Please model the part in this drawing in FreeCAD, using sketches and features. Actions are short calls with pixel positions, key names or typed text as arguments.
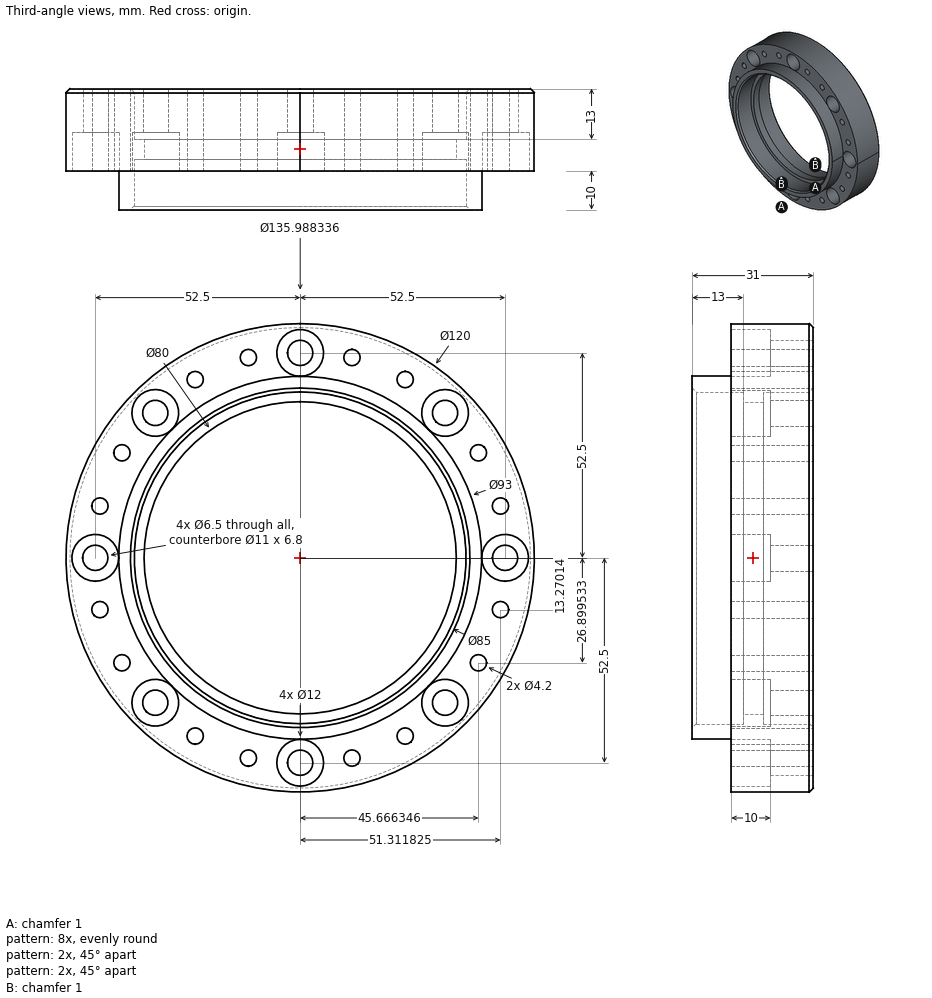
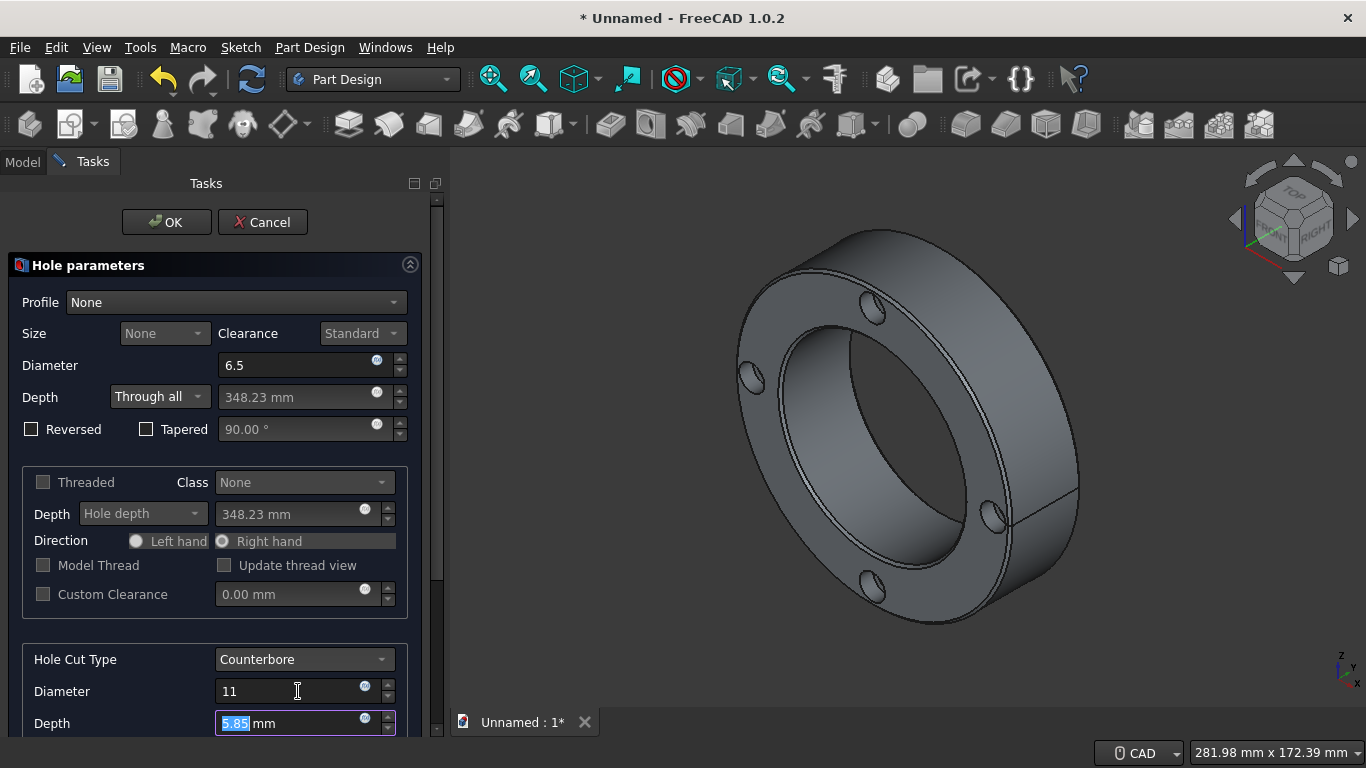
text(6.8)
key(Tab)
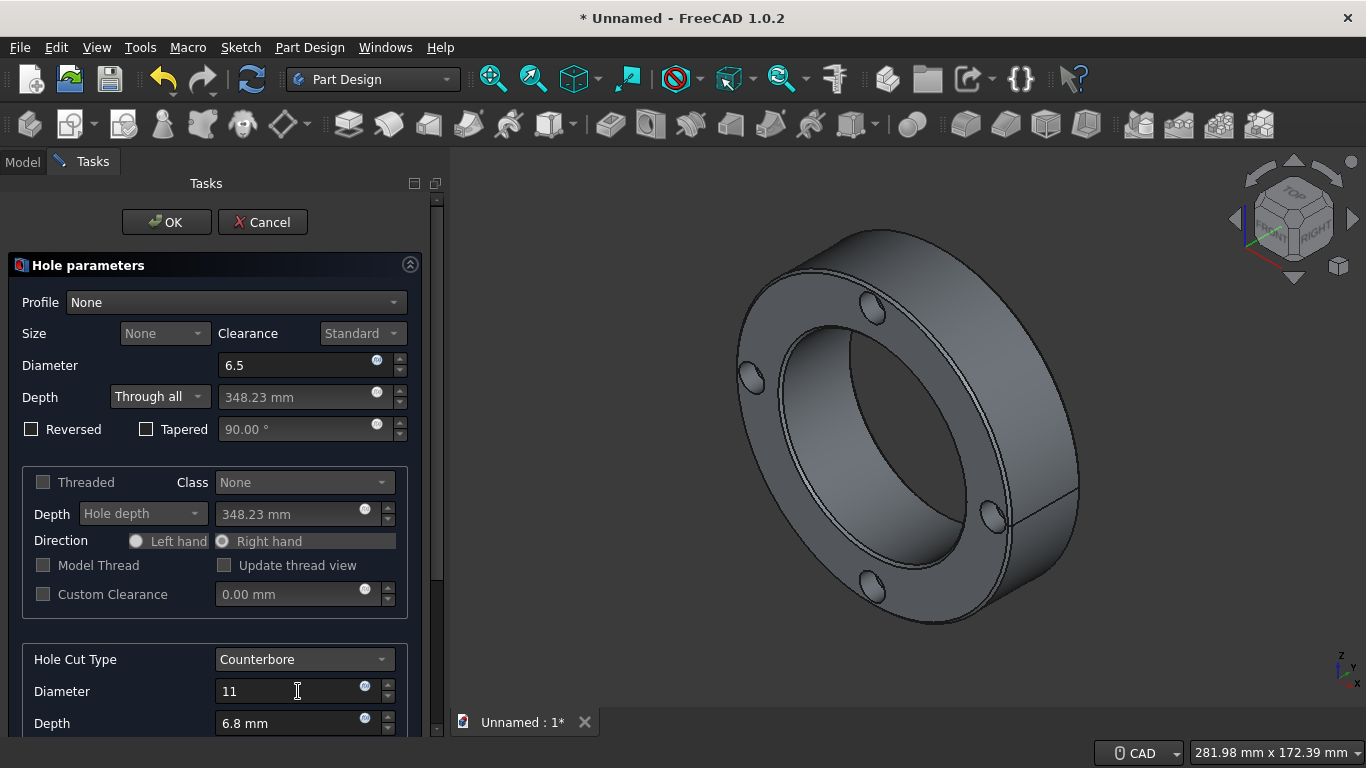
click(167, 222)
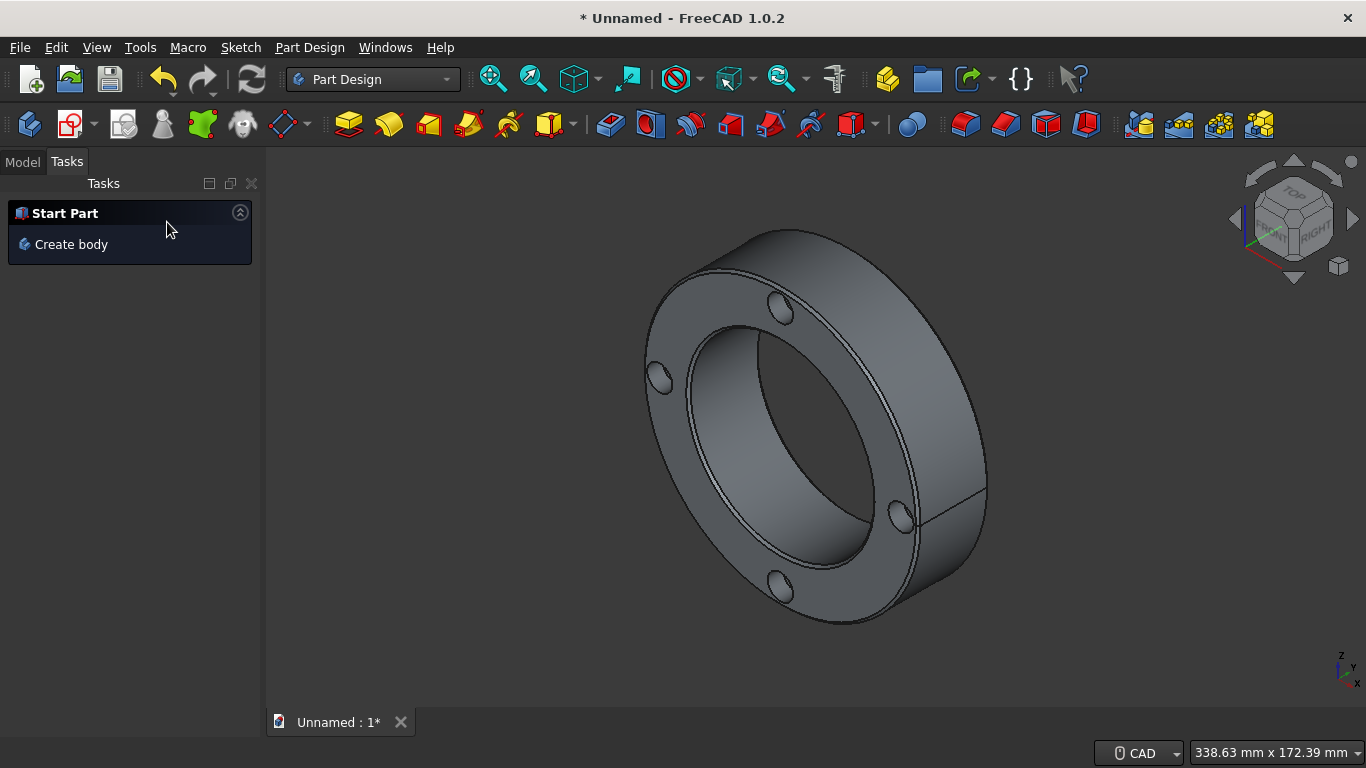
key(4)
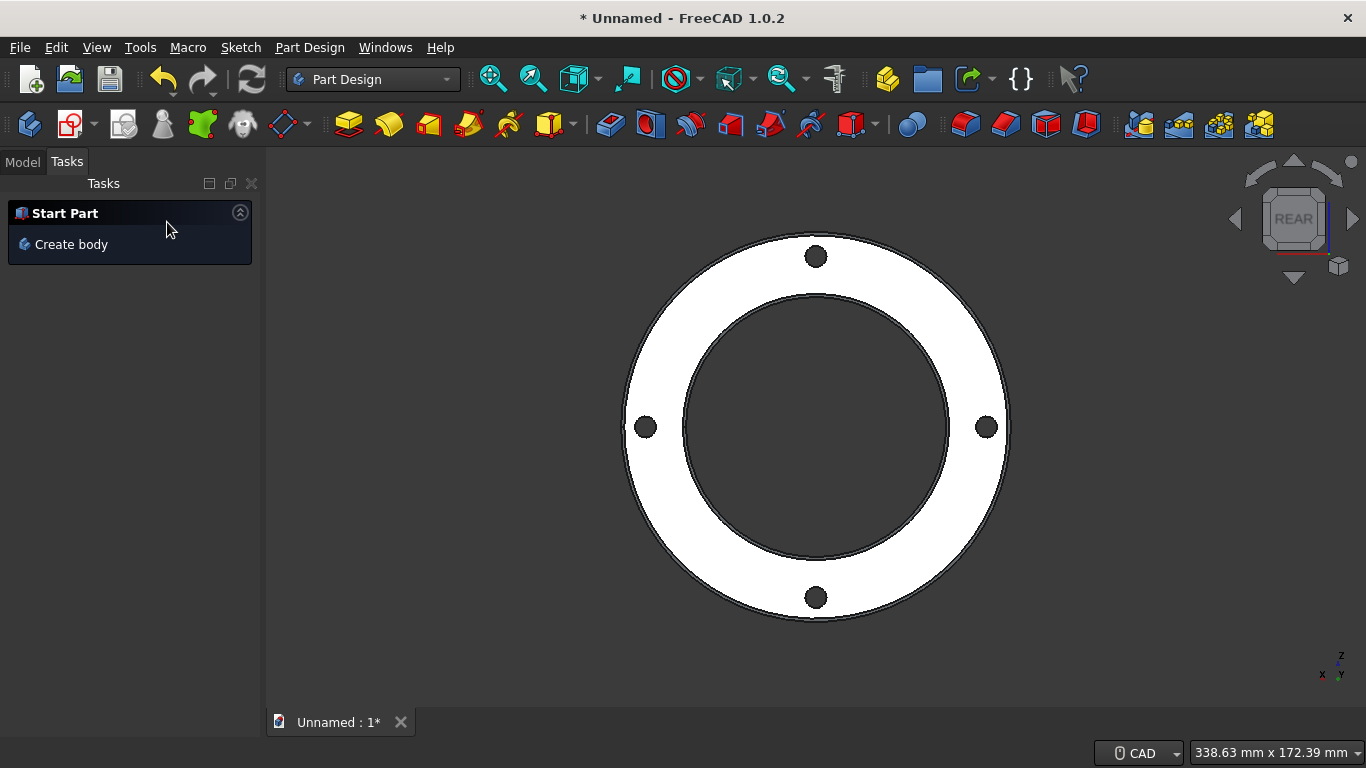
click(926, 316)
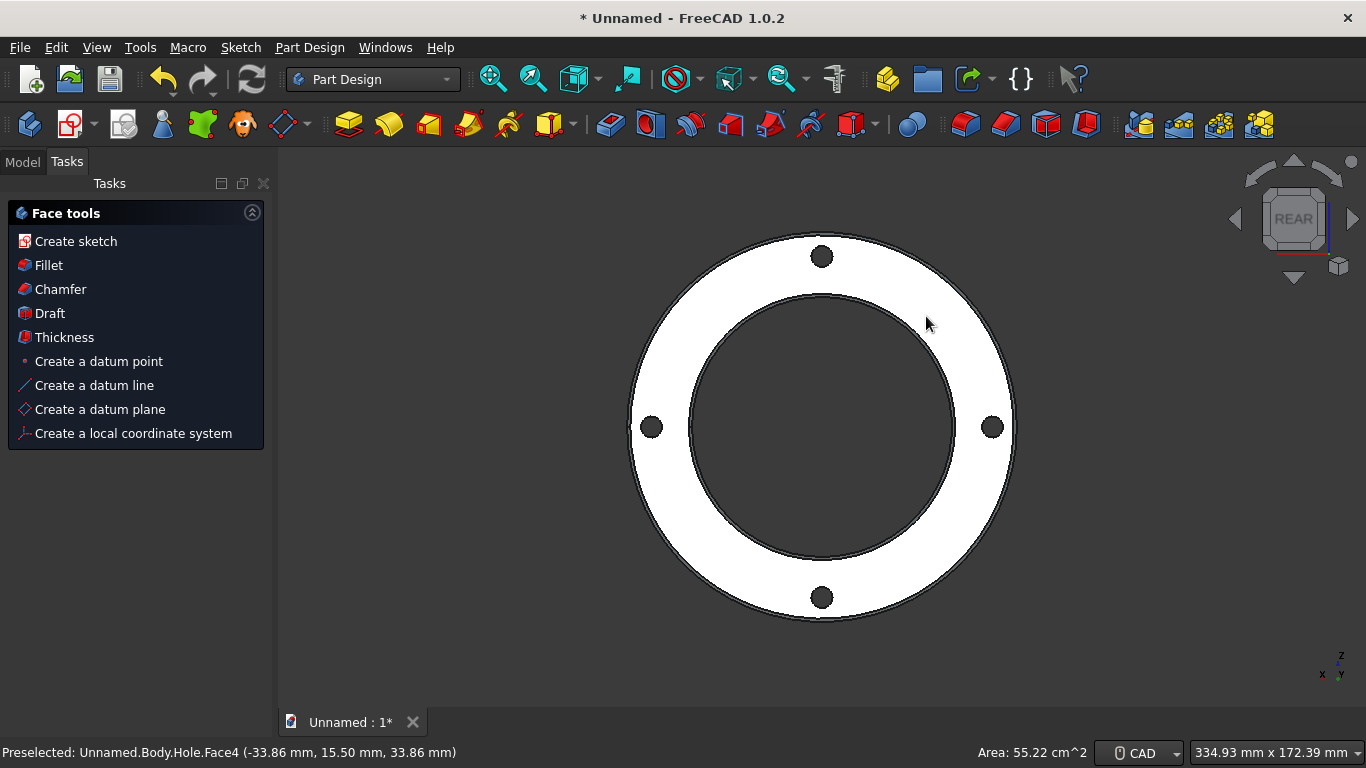
click(70, 124)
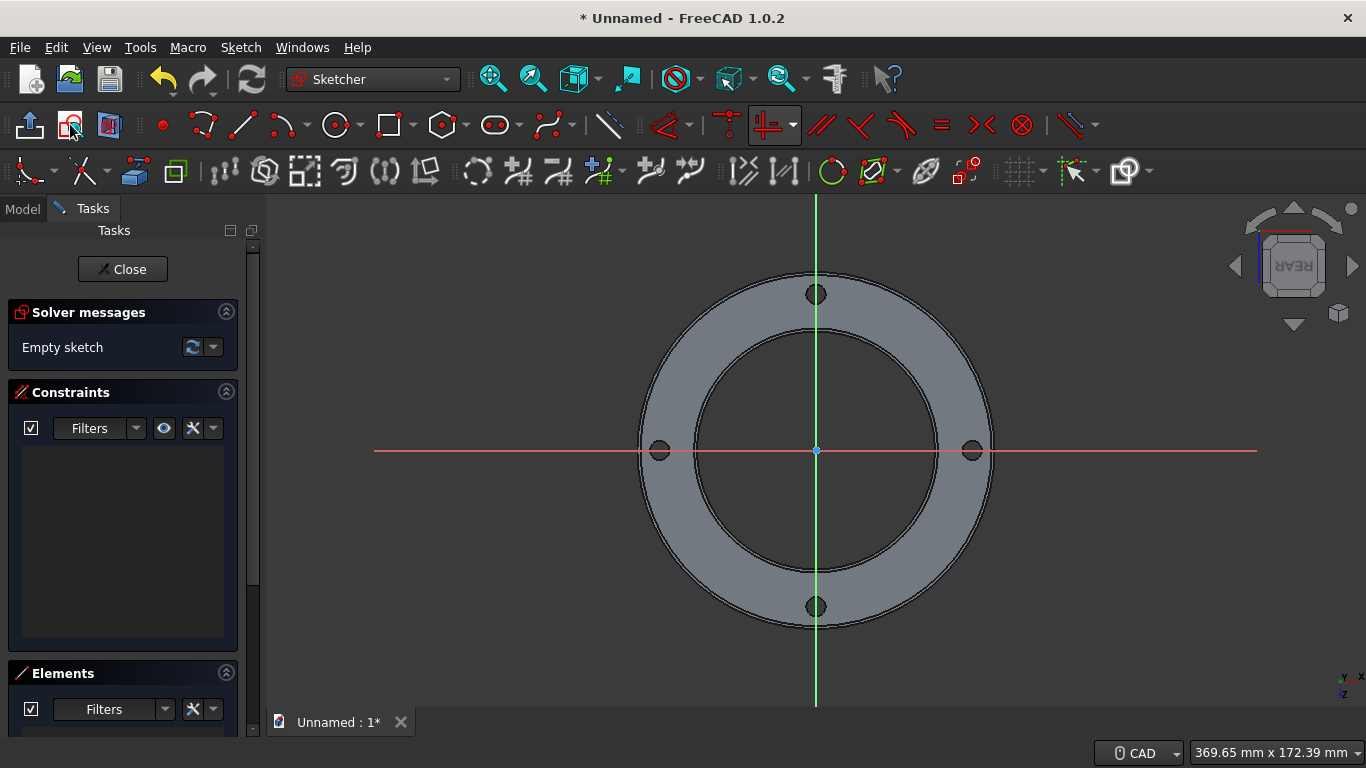
click(336, 126)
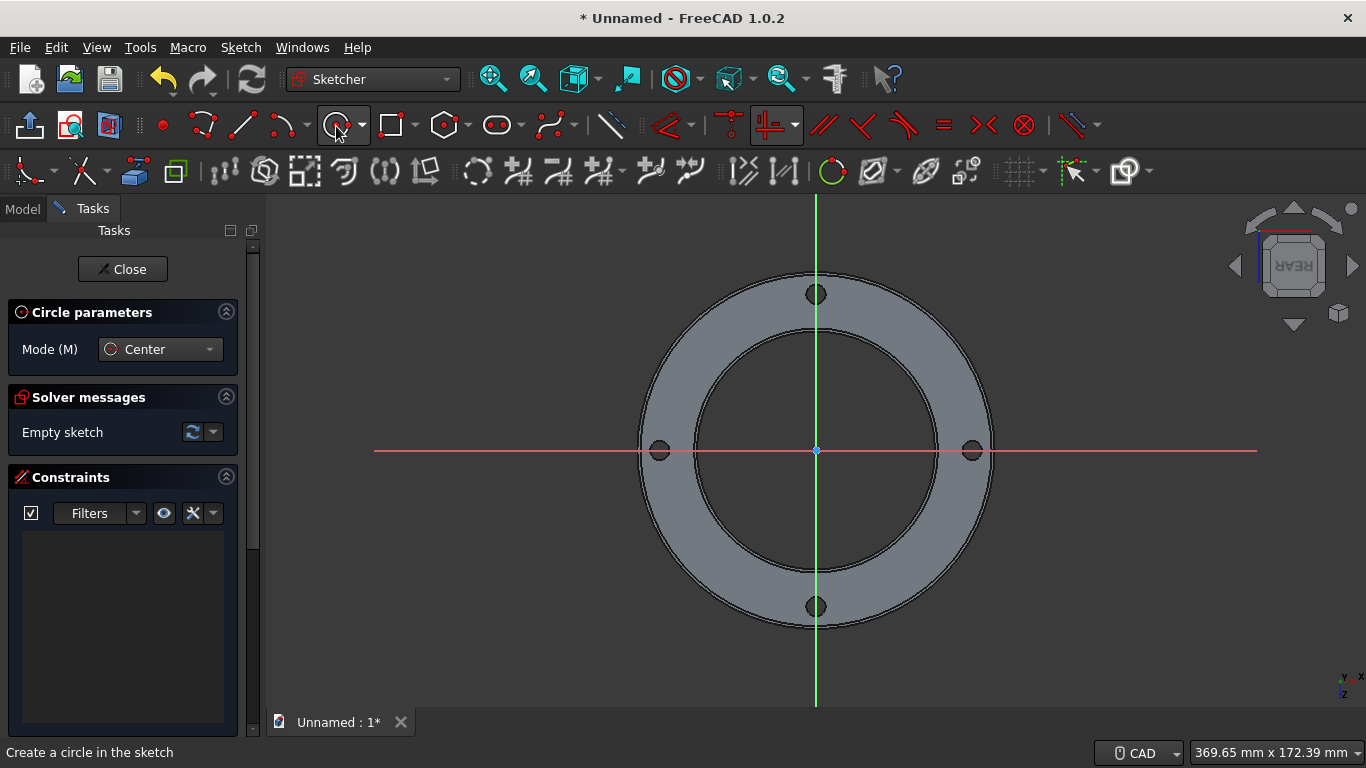
click(816, 451)
move(905, 361)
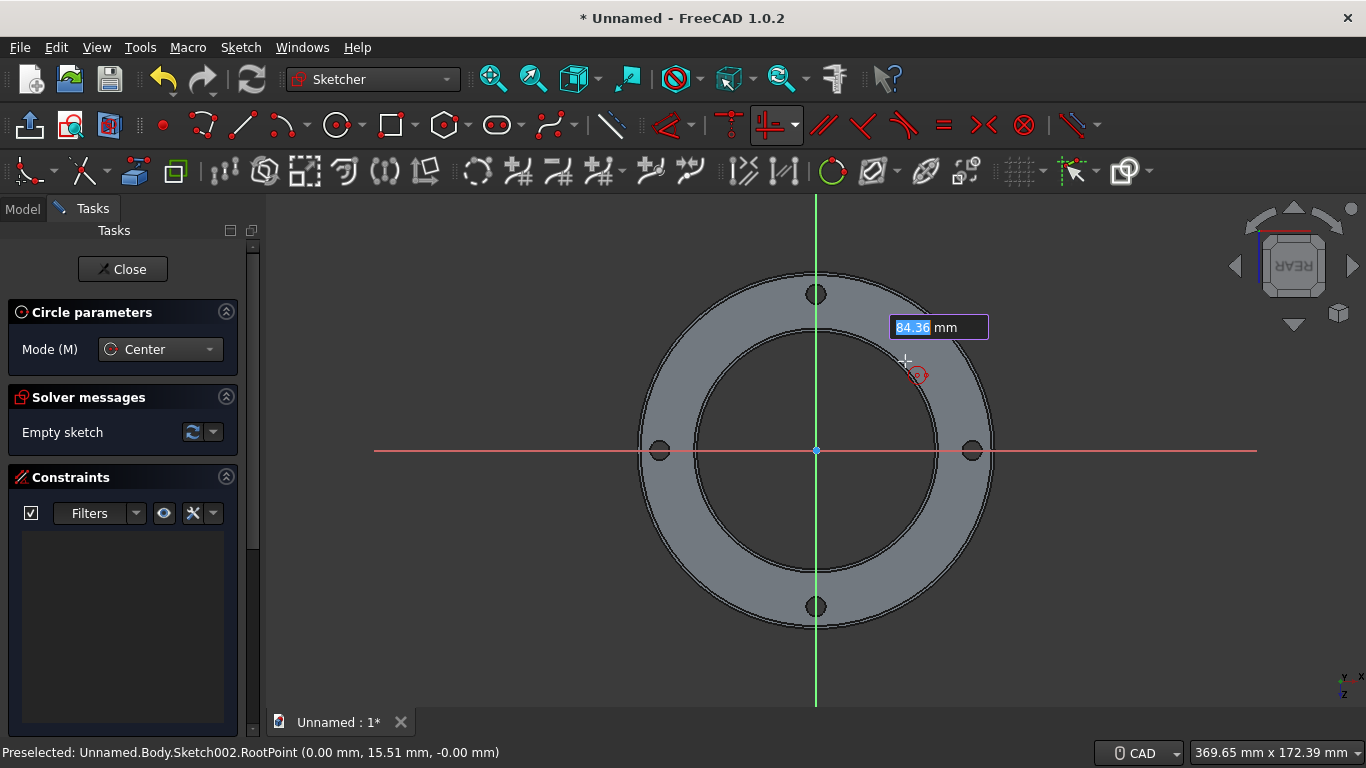
text(85)
key(Return)
key(Escape)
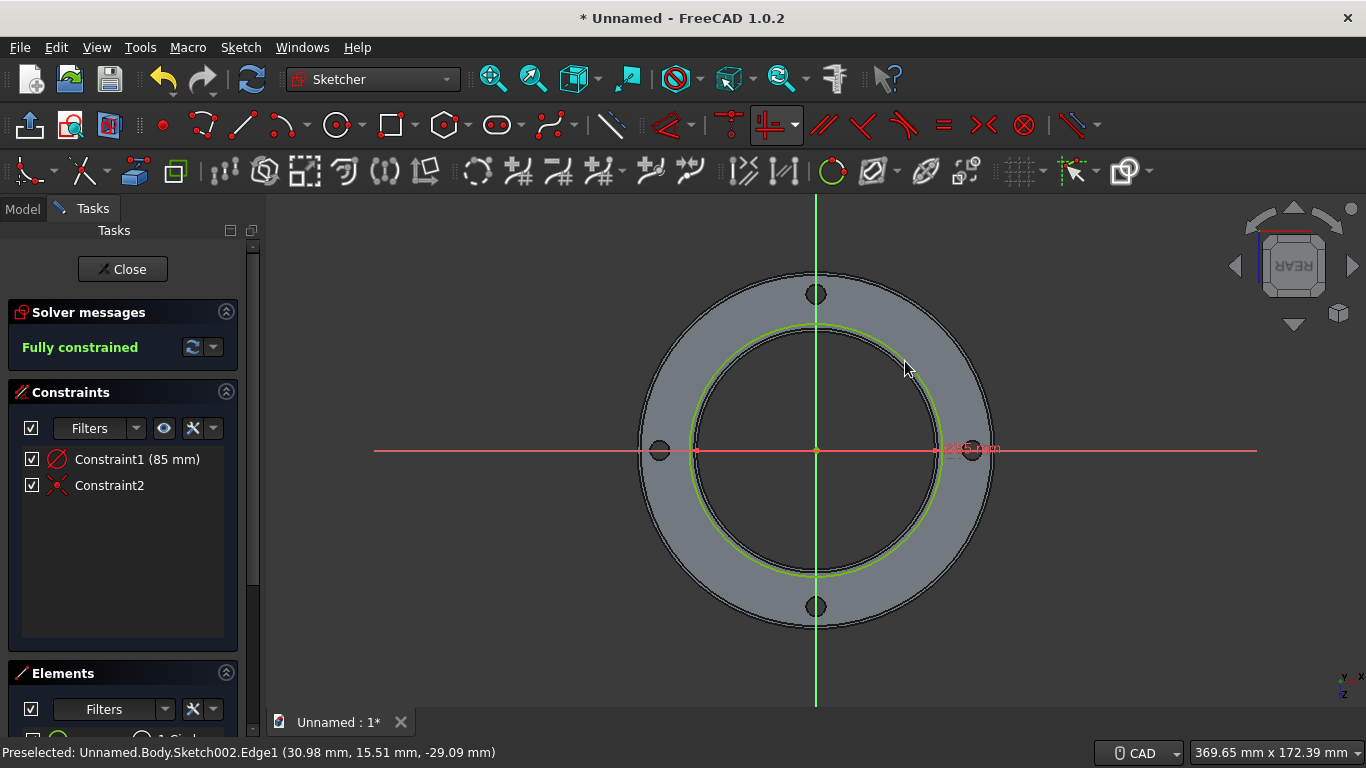
click(123, 269)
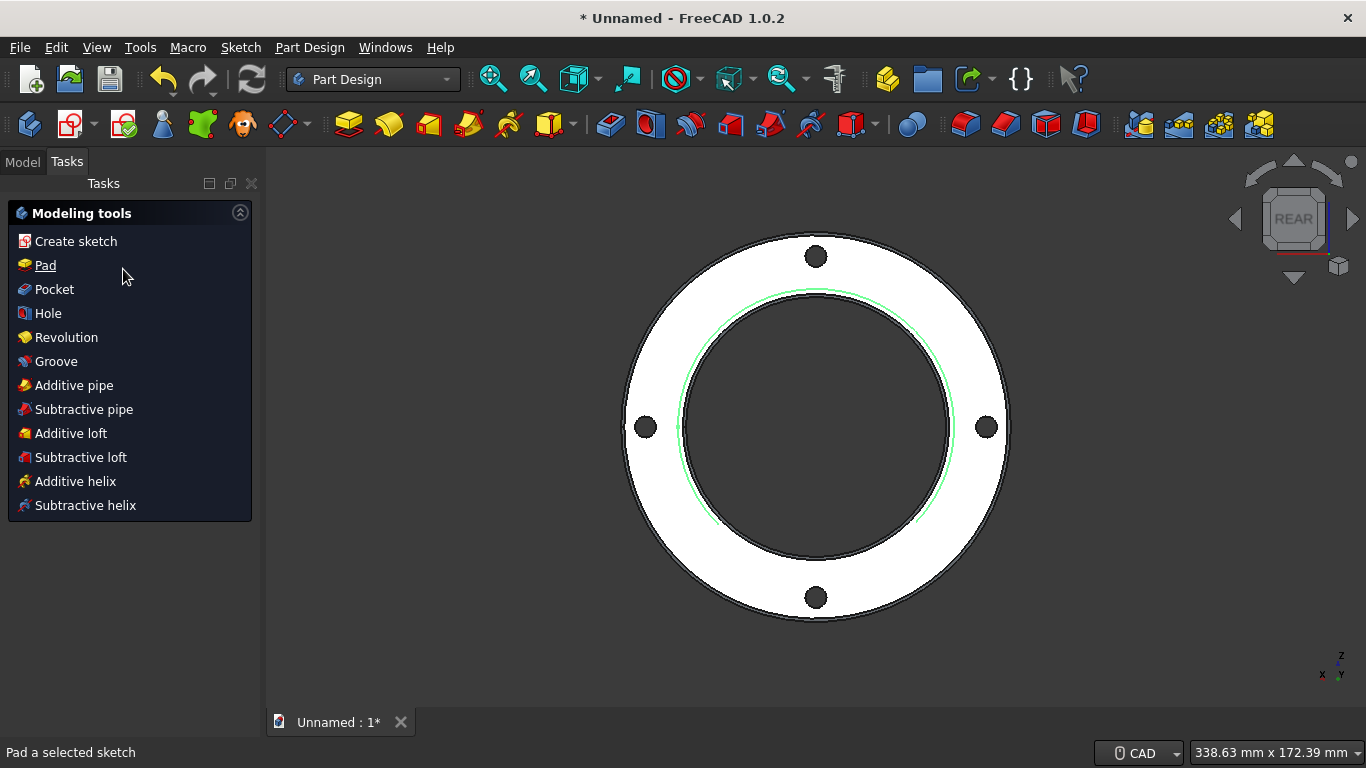
click(612, 124)